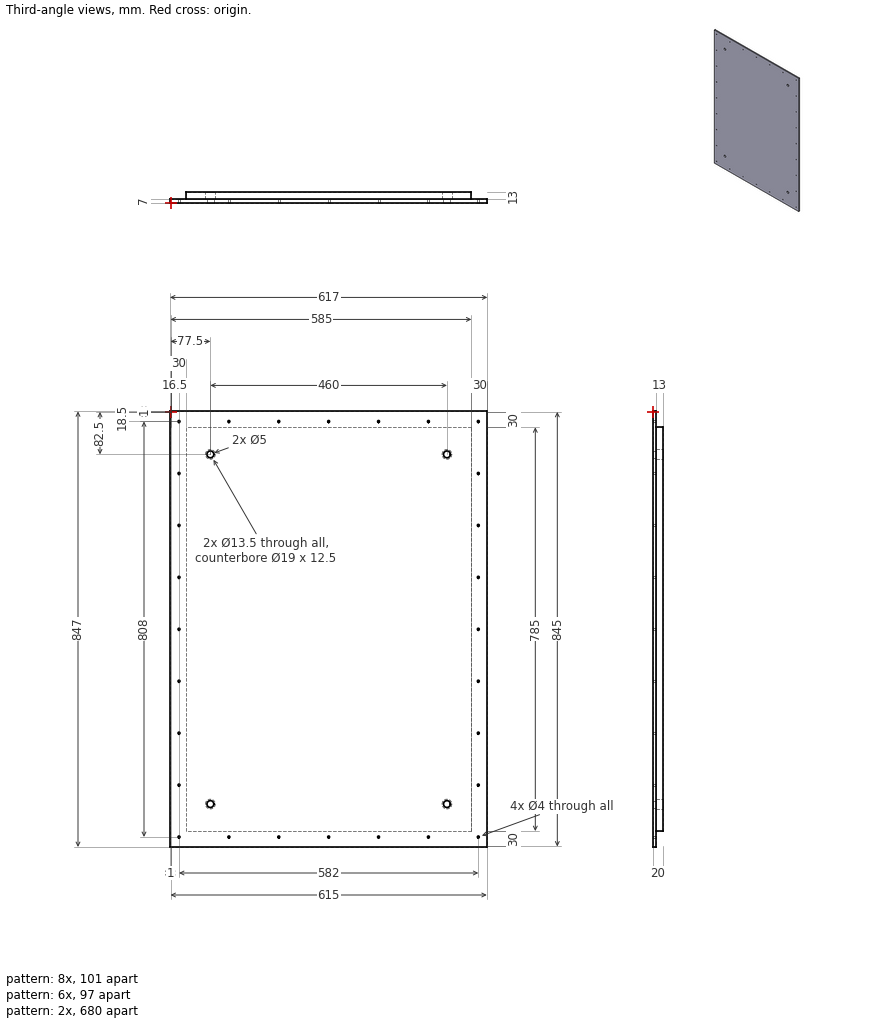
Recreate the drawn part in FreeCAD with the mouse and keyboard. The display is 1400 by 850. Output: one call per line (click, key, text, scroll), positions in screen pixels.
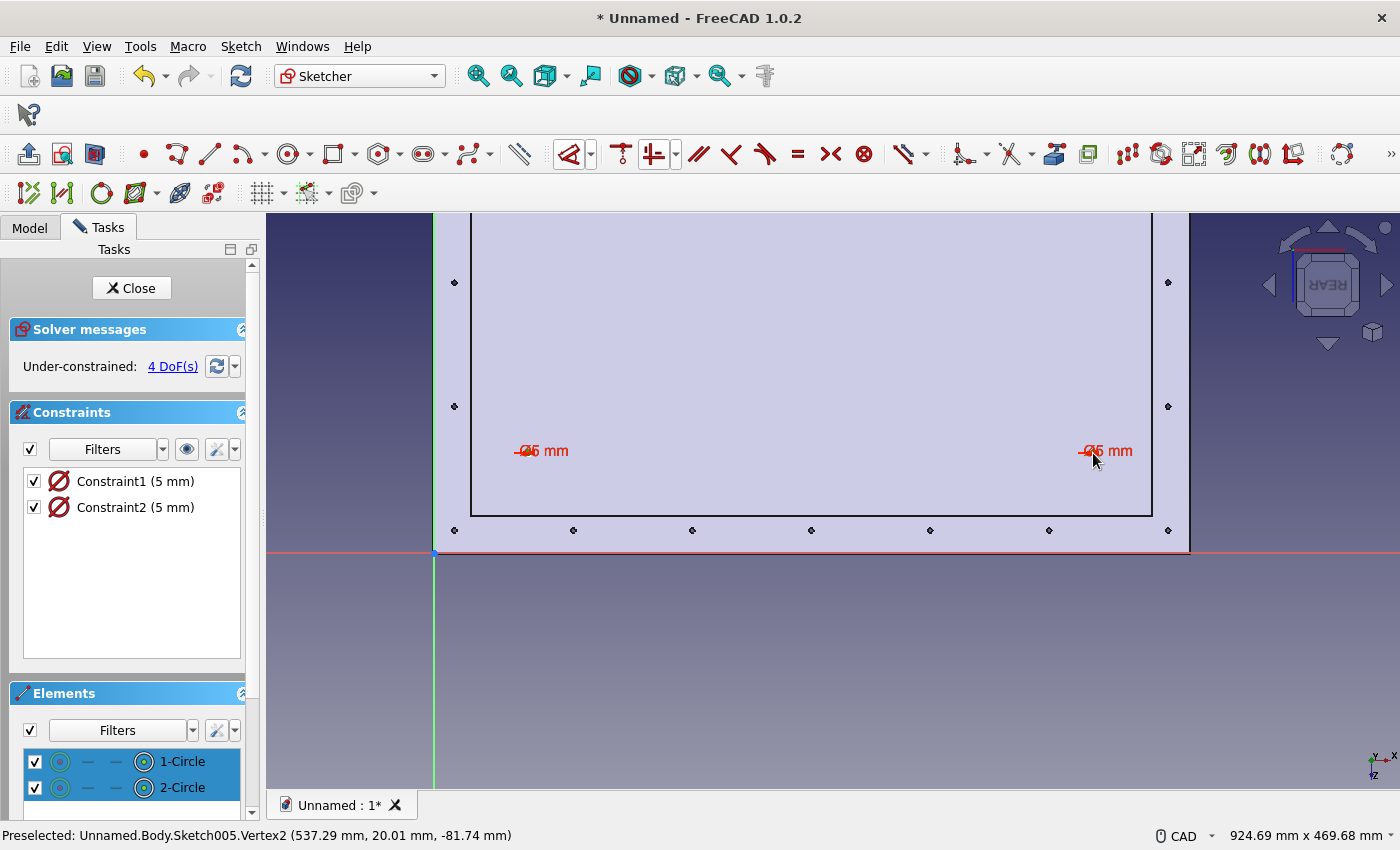
click(676, 154)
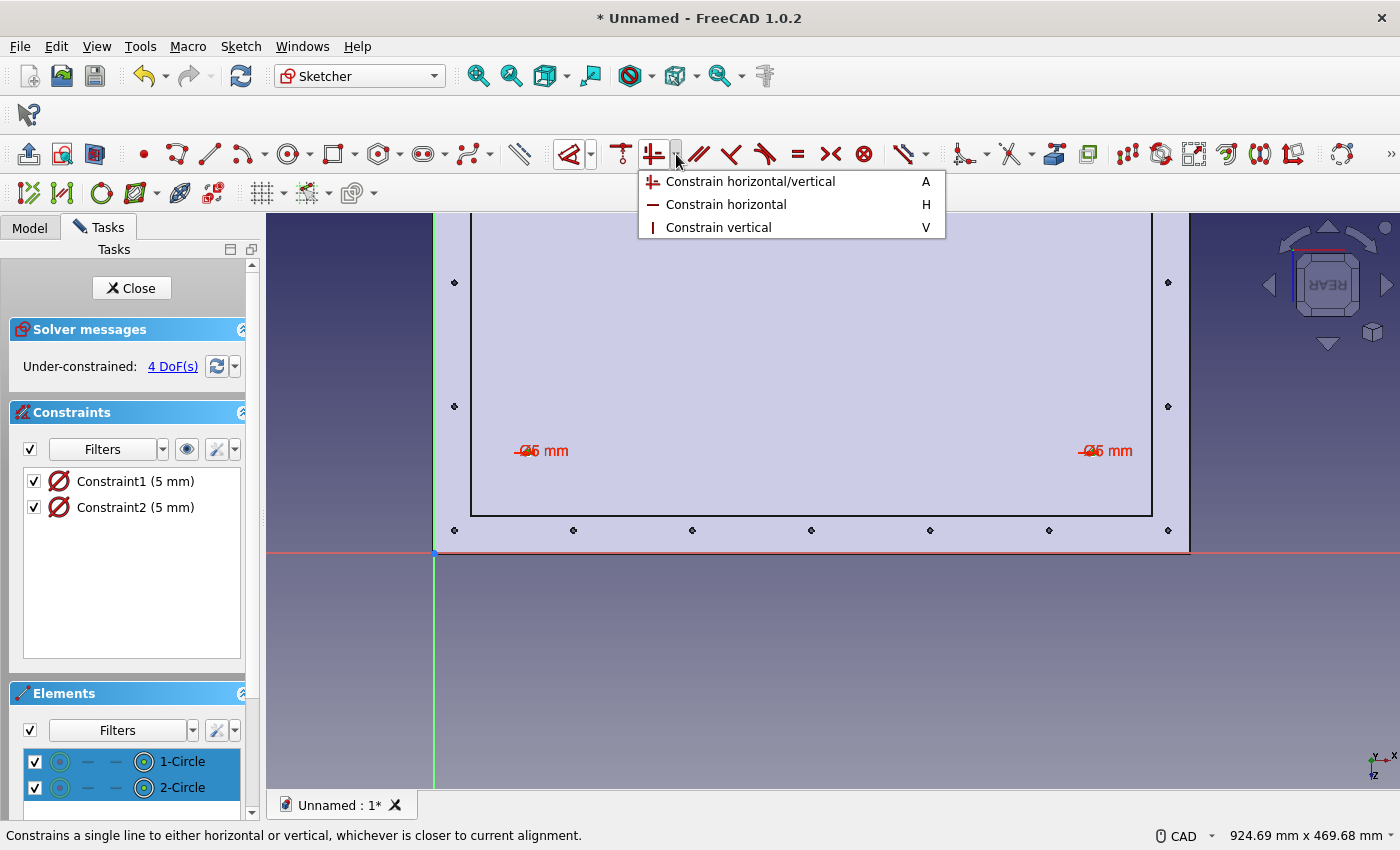
click(792, 204)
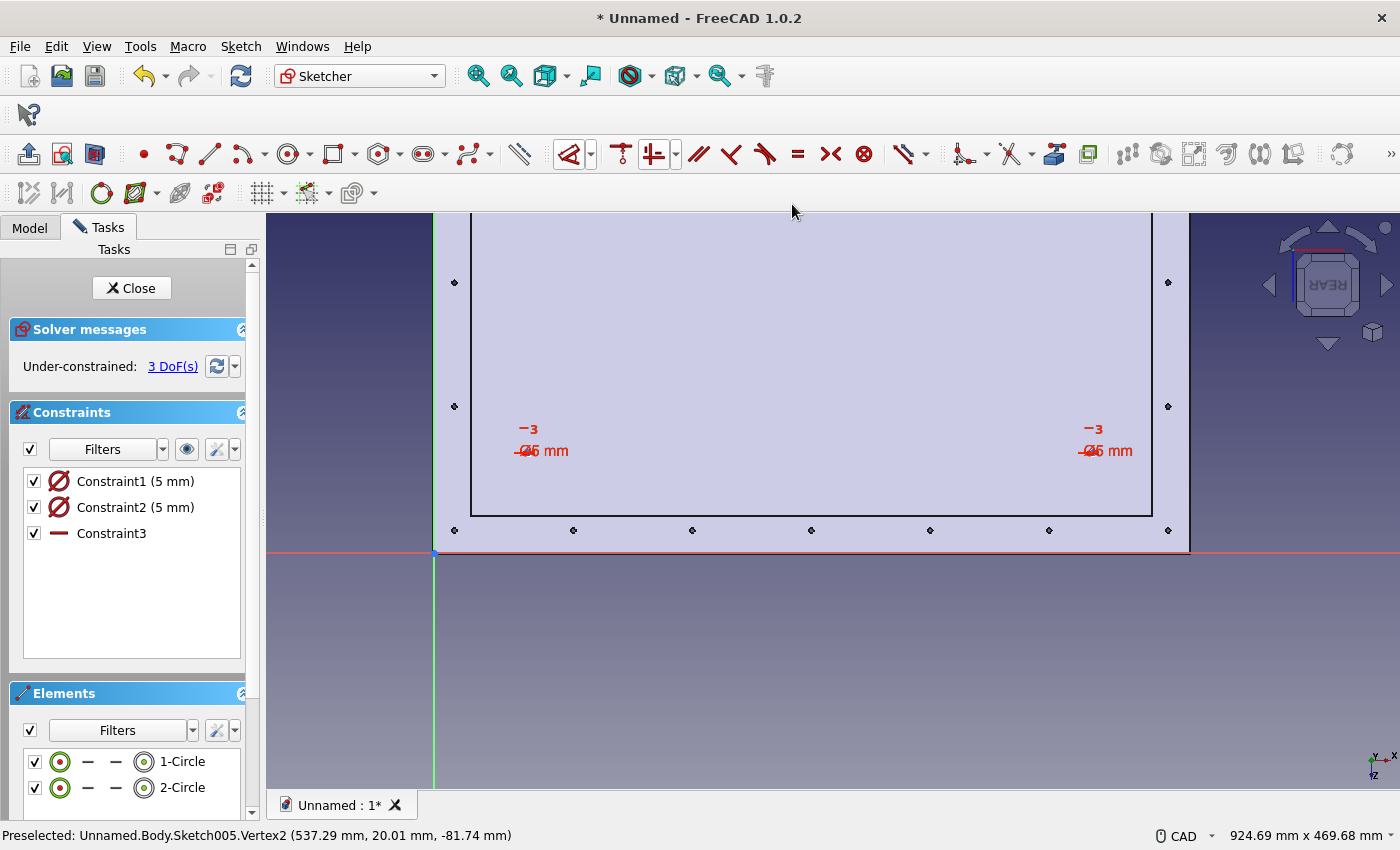
click(529, 453)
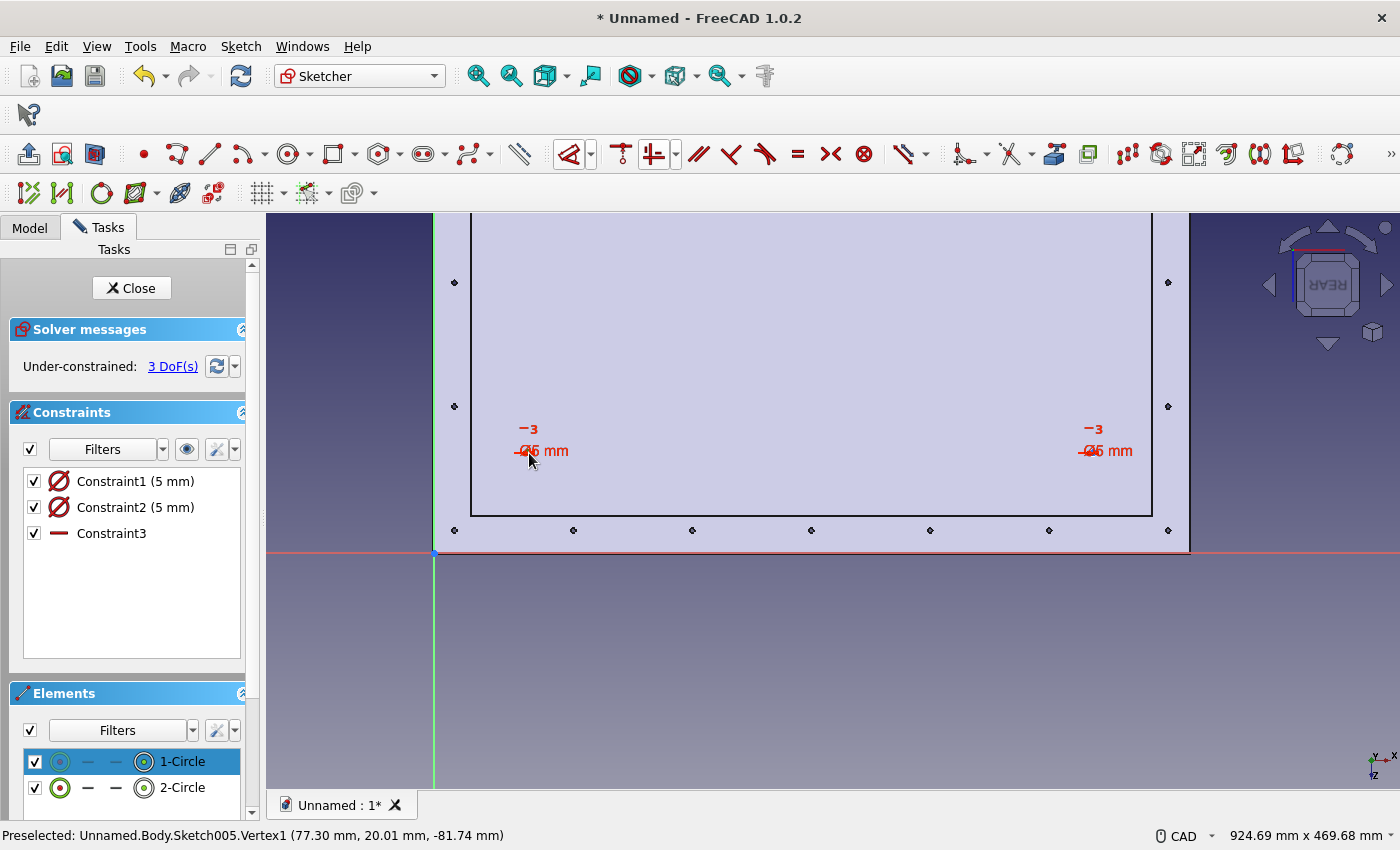
key(l)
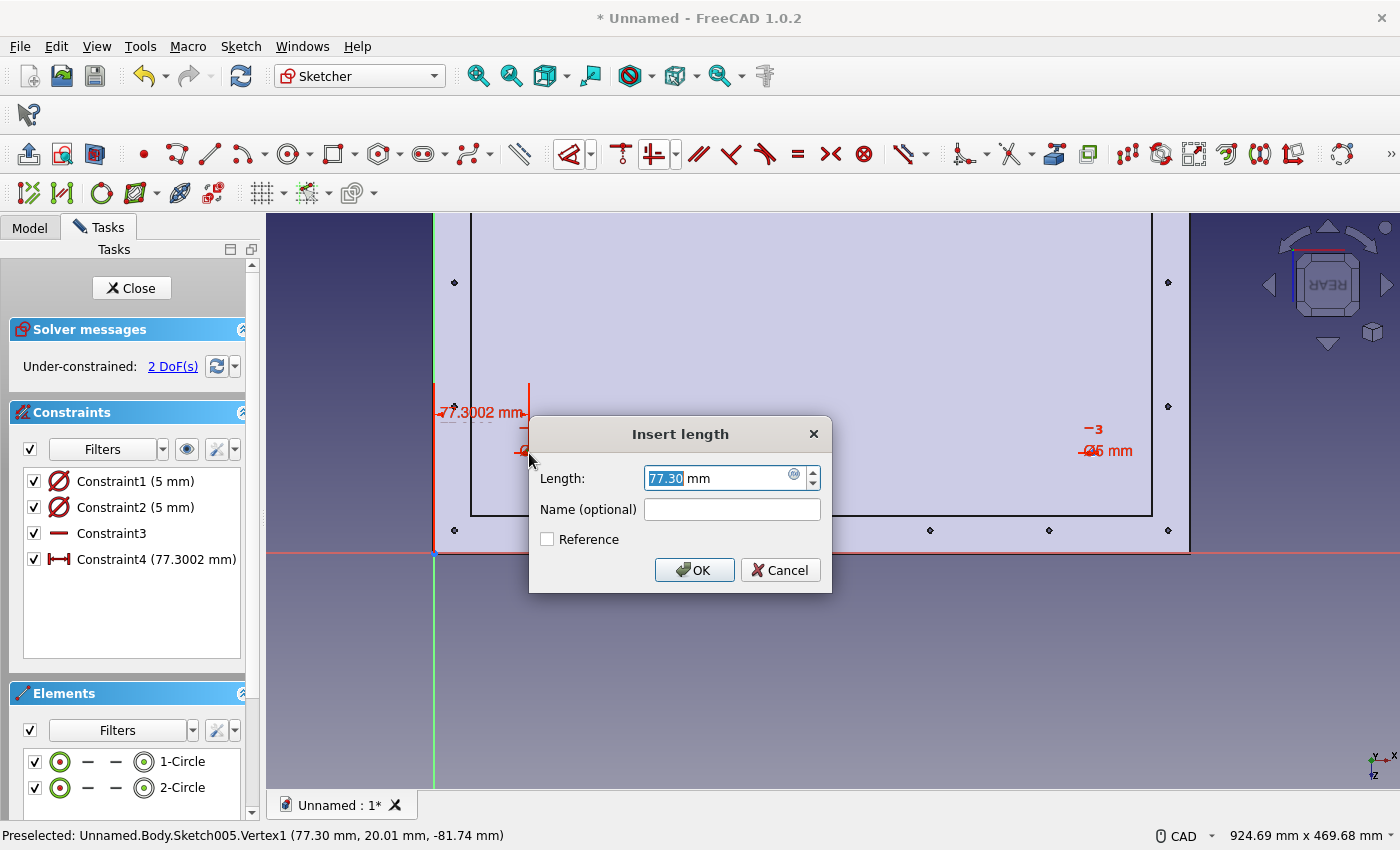
text(77.5)
key(Return)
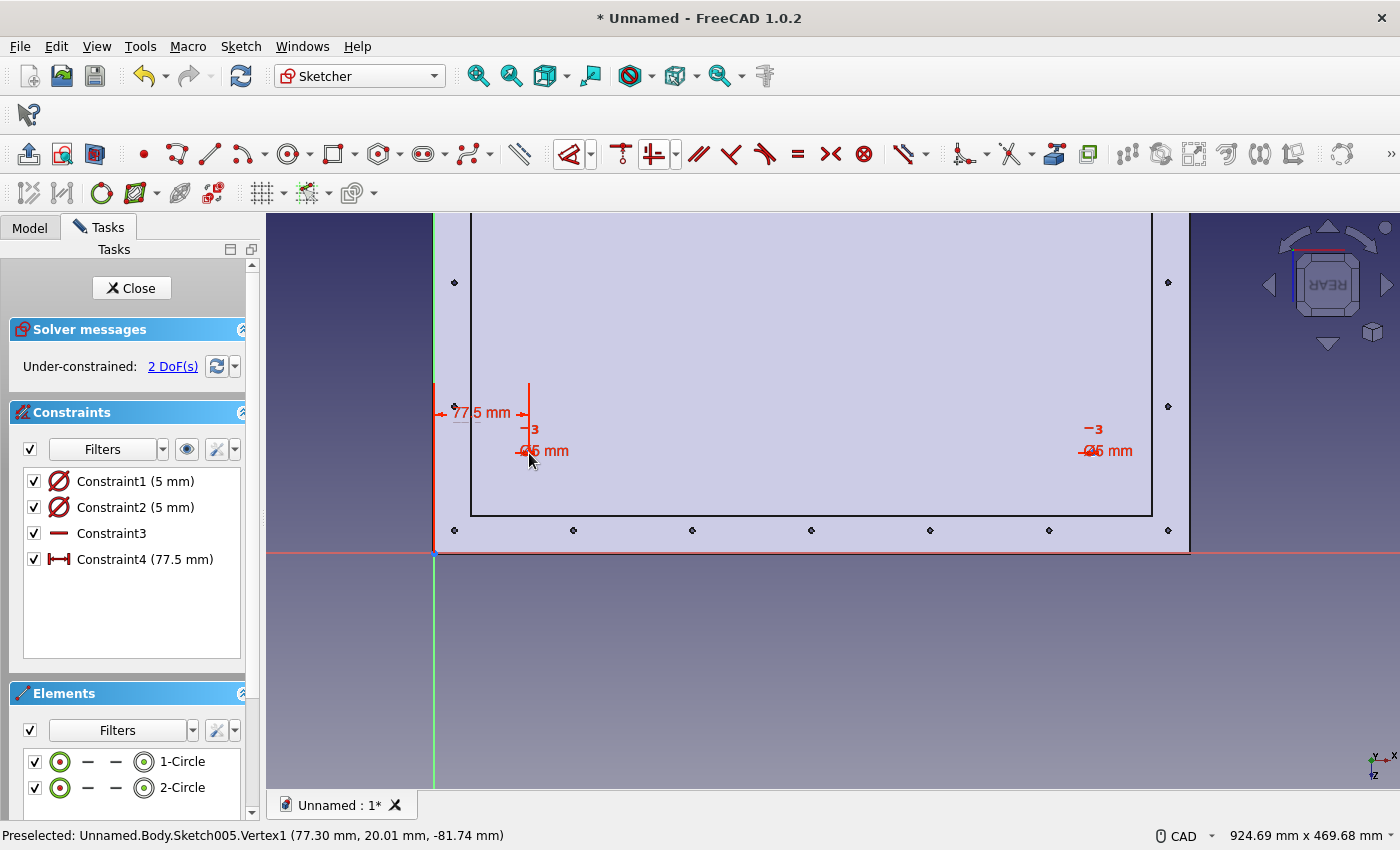
click(529, 453)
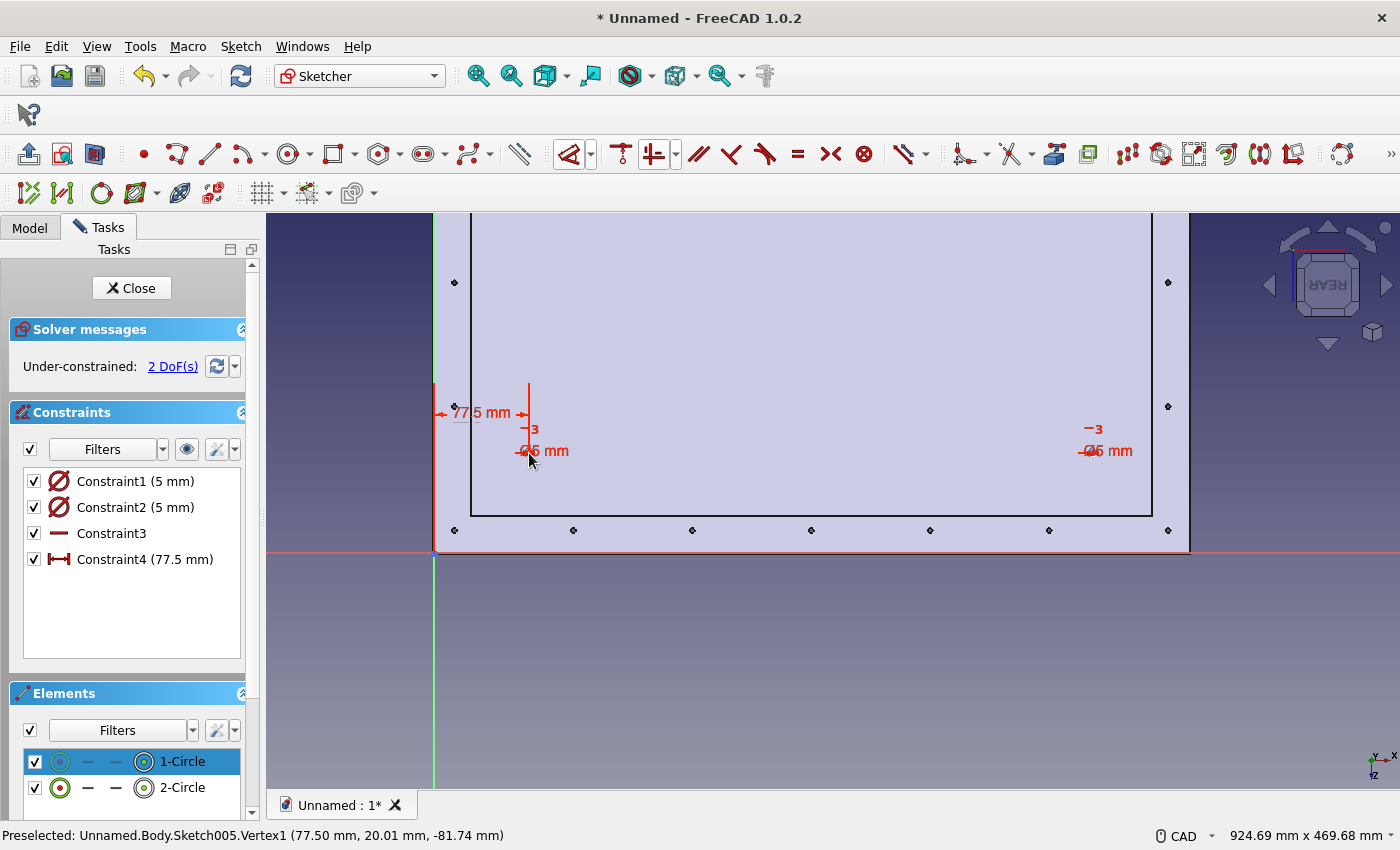
key(i)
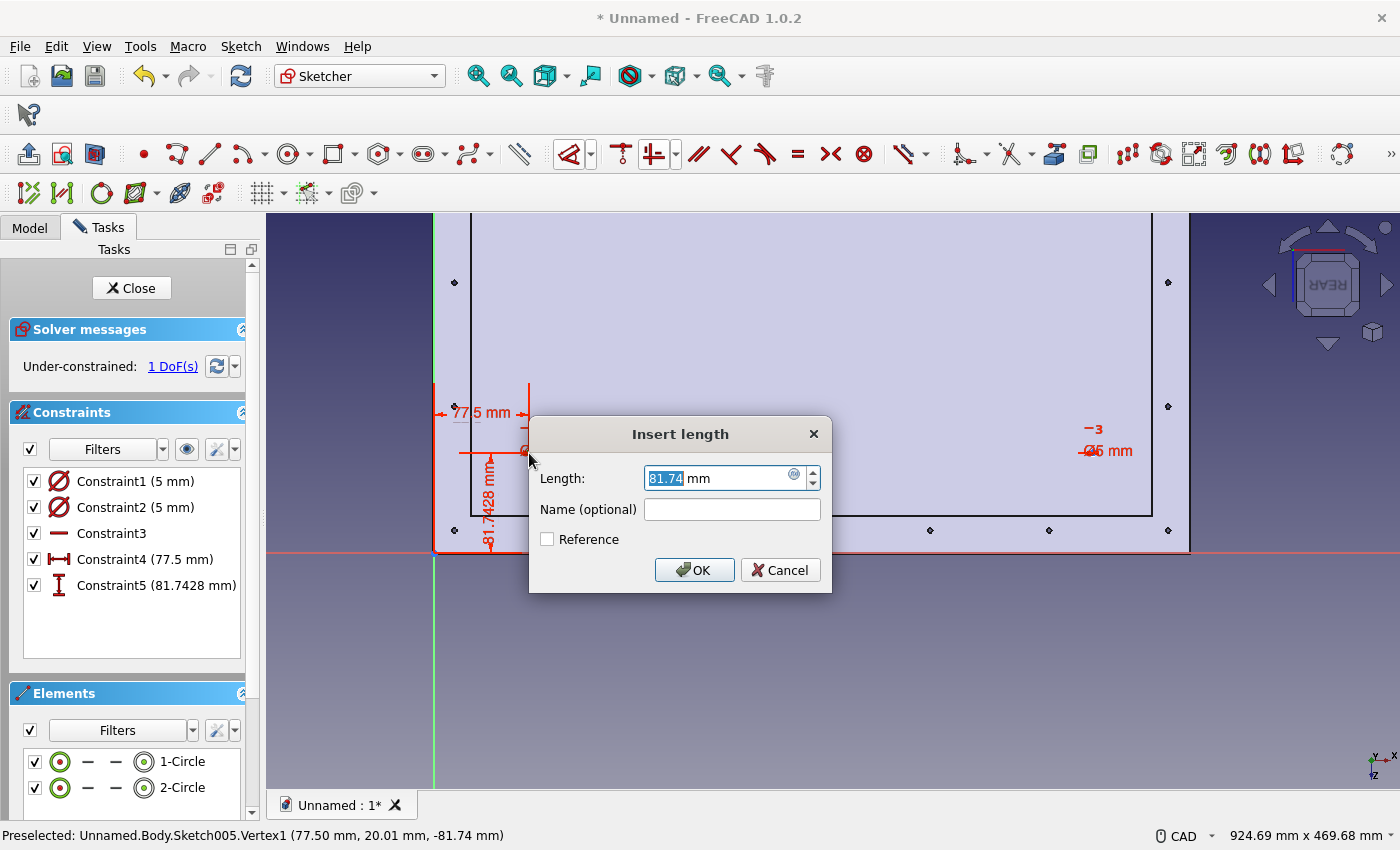
text(82.5)
key(Return)